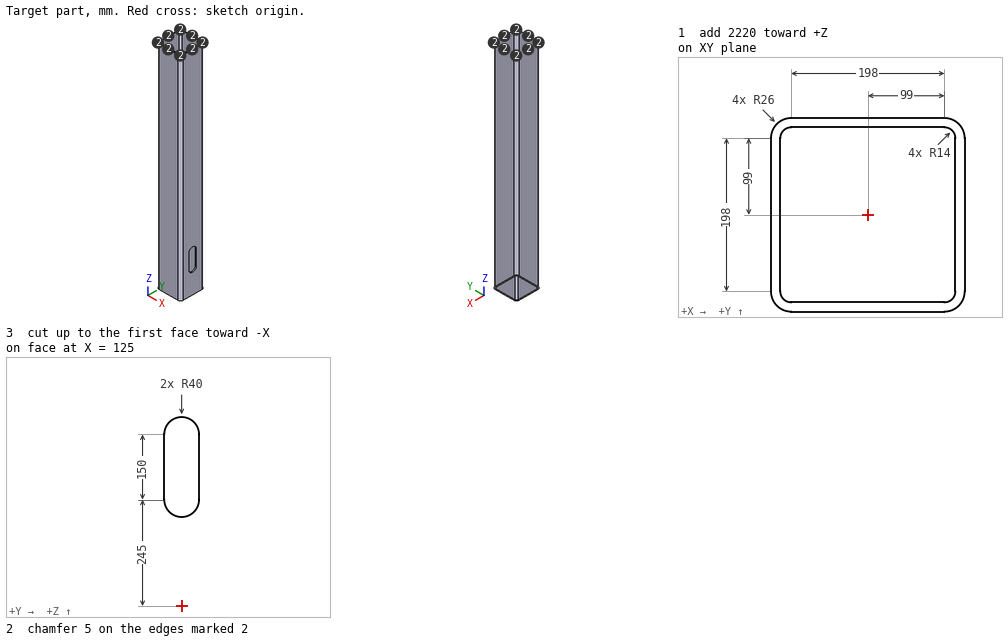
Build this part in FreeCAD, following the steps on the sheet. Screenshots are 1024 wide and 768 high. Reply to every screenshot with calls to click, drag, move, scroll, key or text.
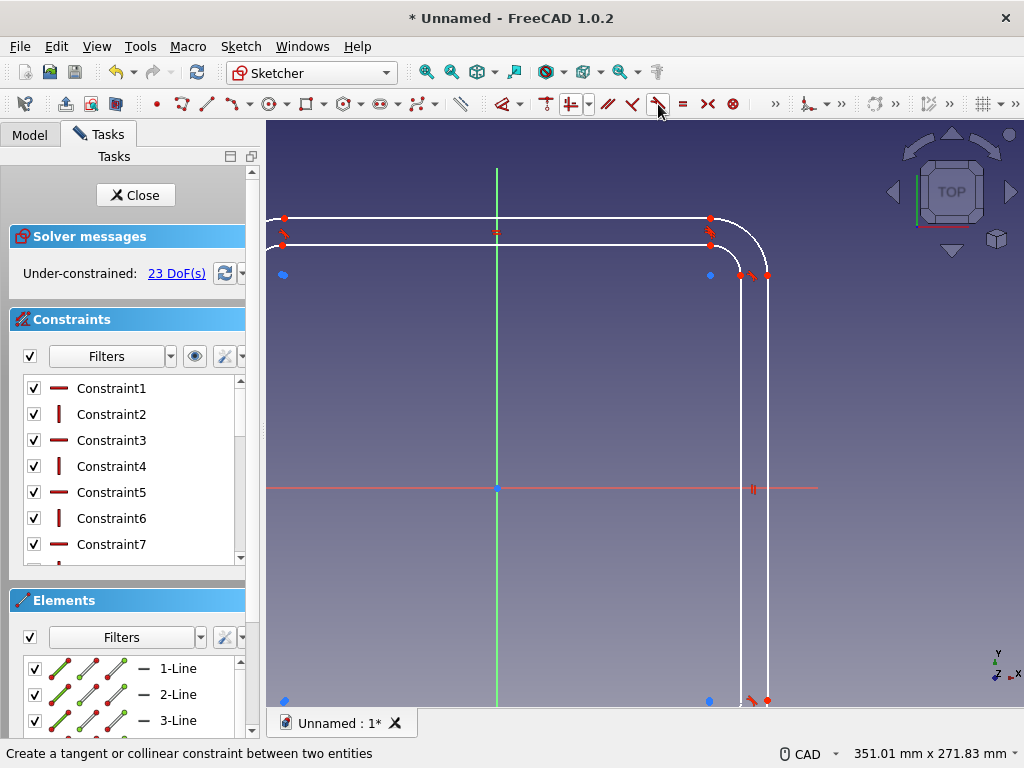
click(411, 245)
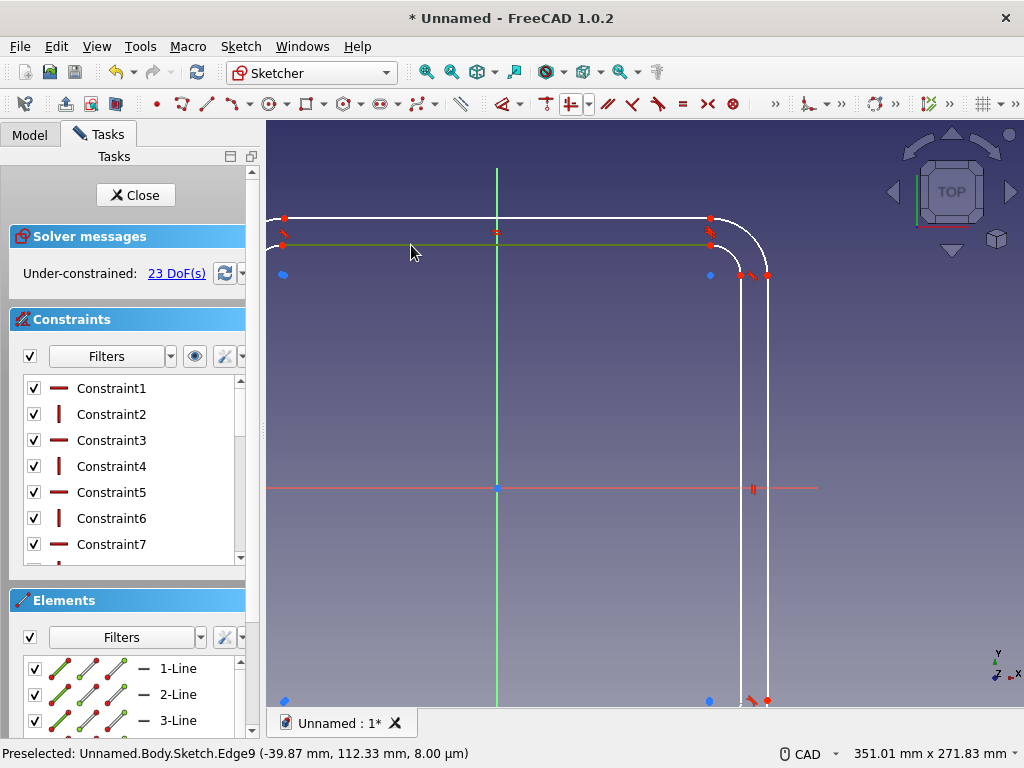
scroll(738, 262, down, 2)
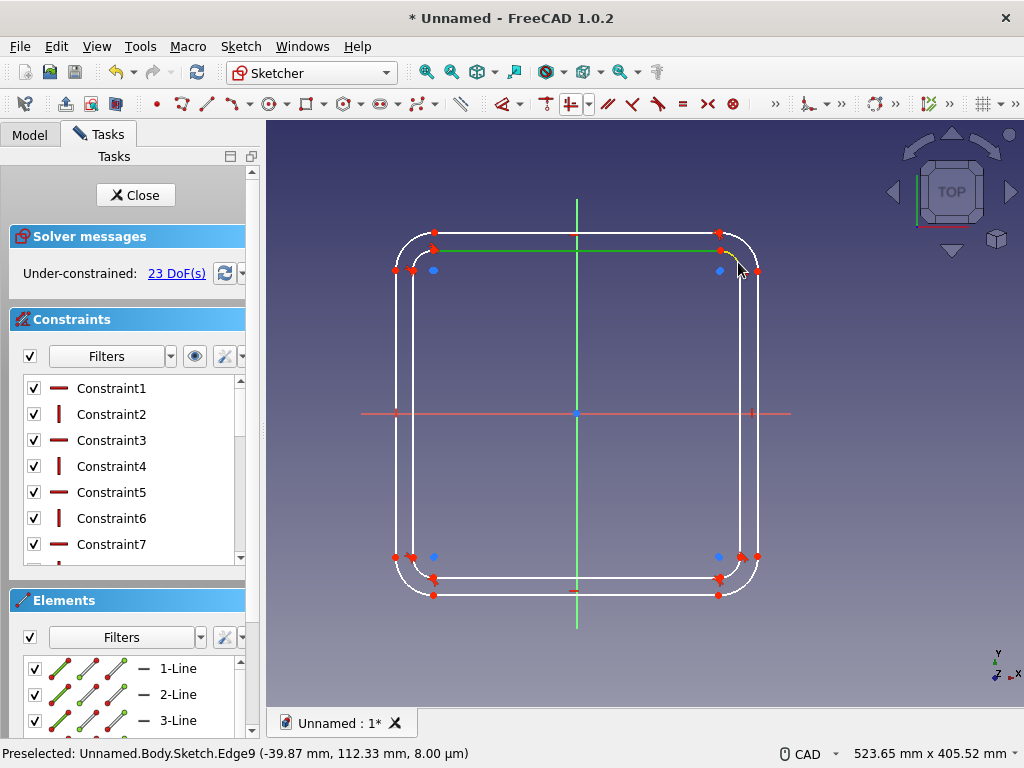
scroll(424, 253, up, 2)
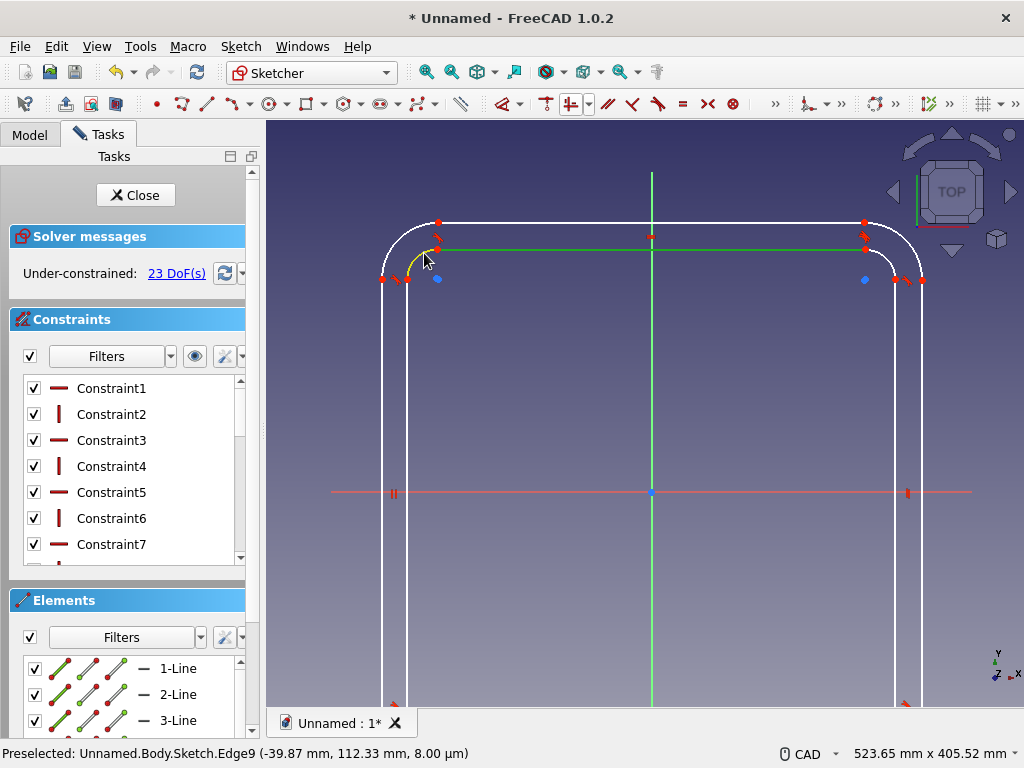
click(424, 253)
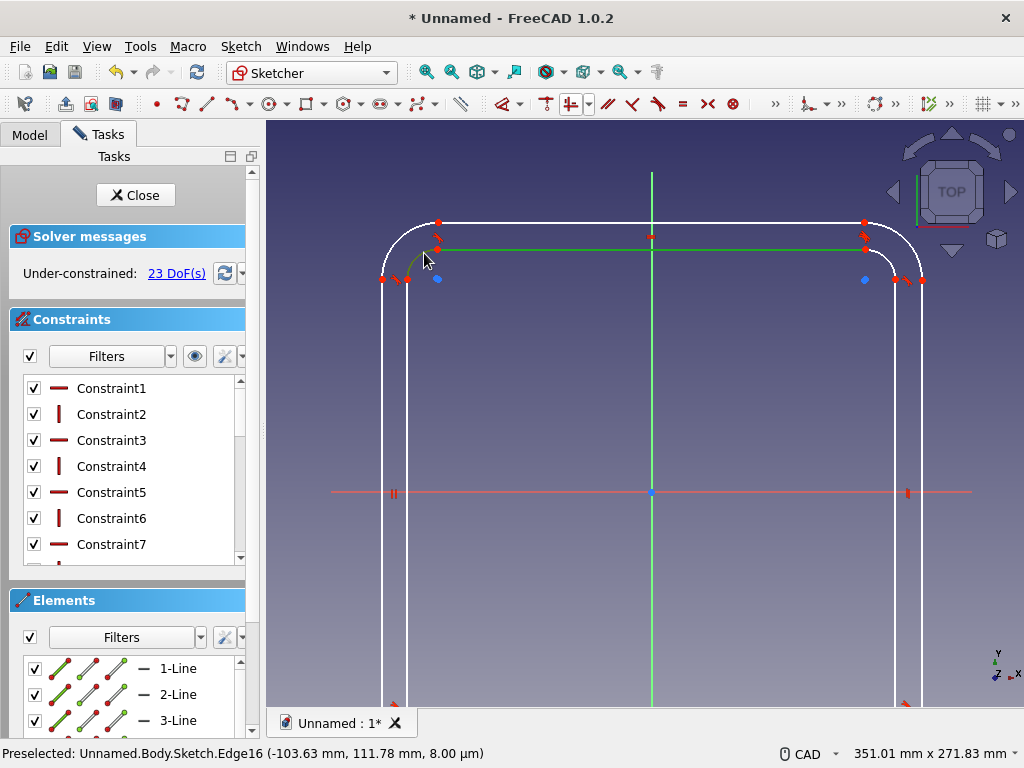
click(658, 104)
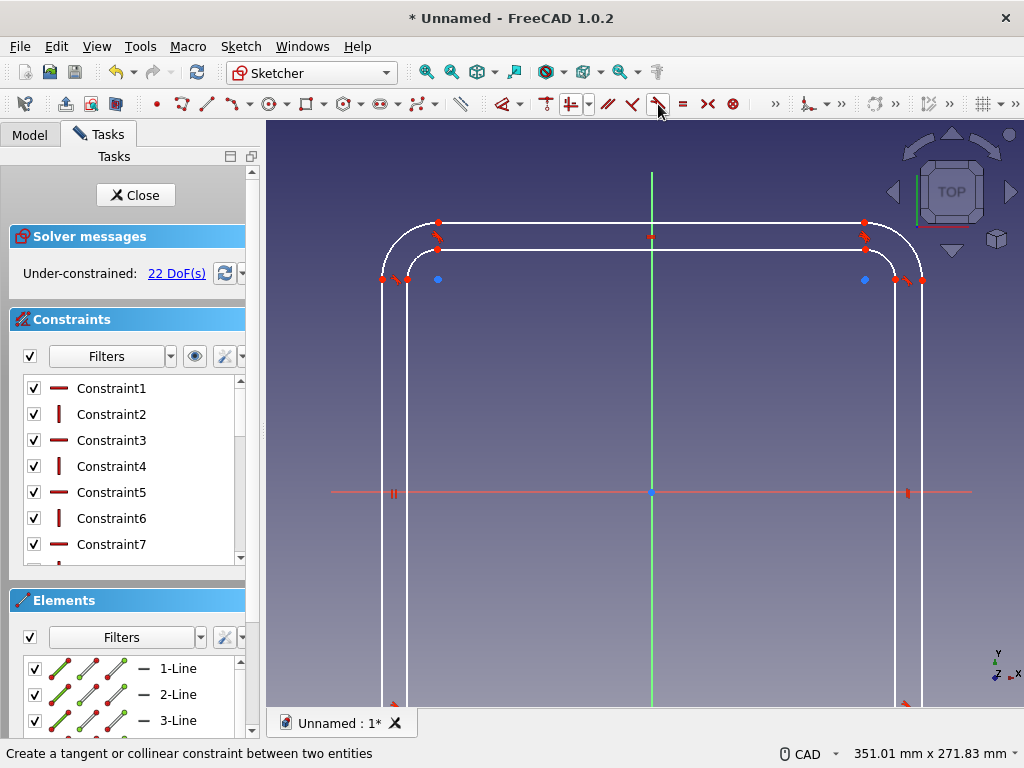
scroll(424, 253, down, 2)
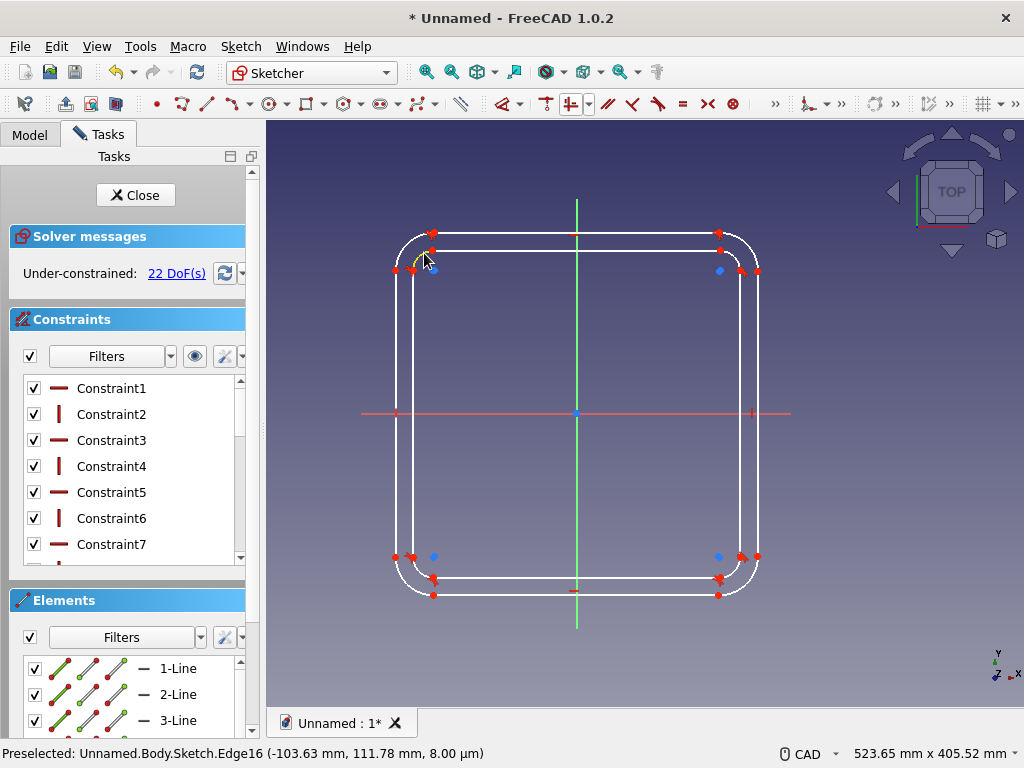
click(740, 357)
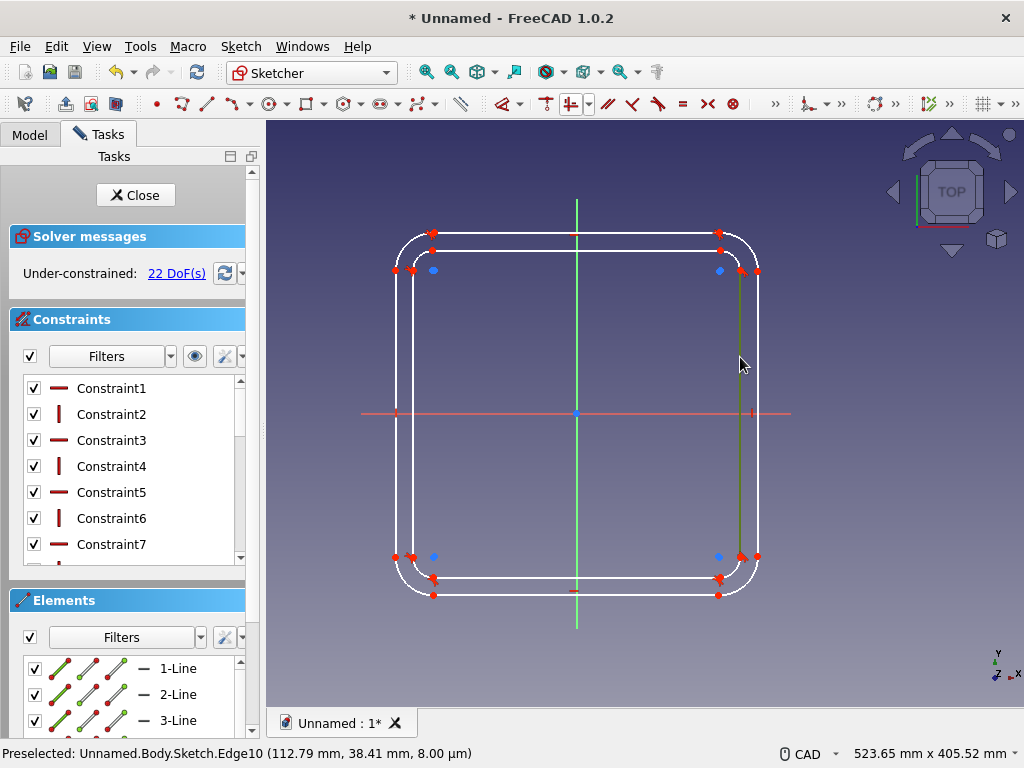
scroll(738, 262, up, 2)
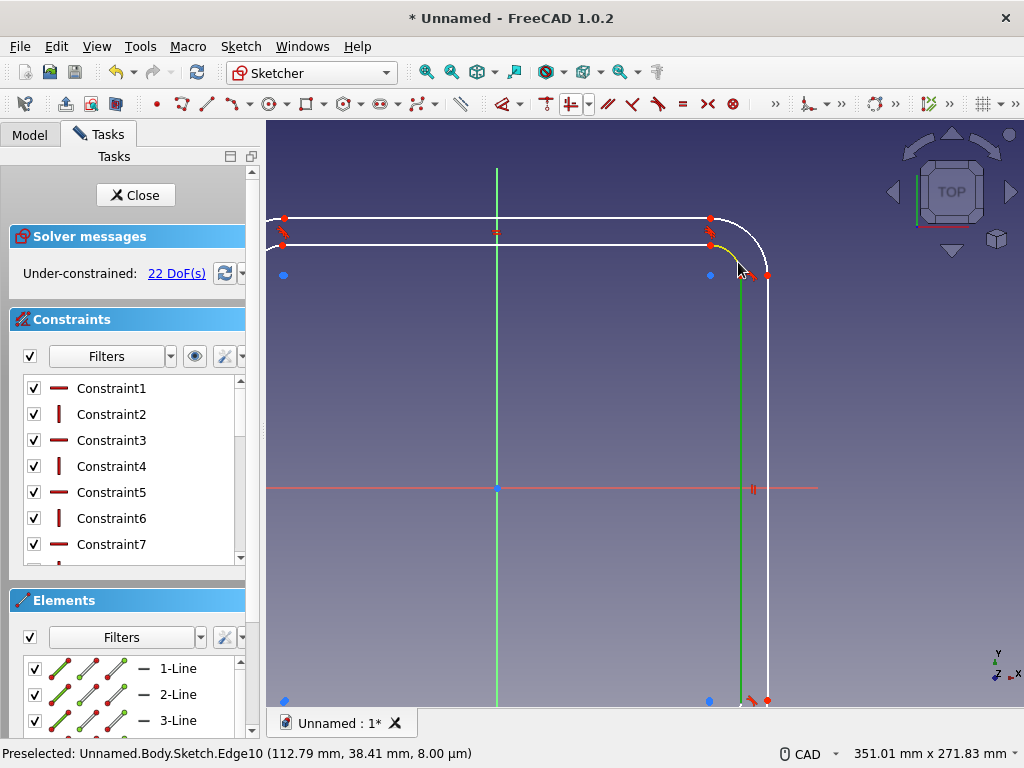
click(737, 262)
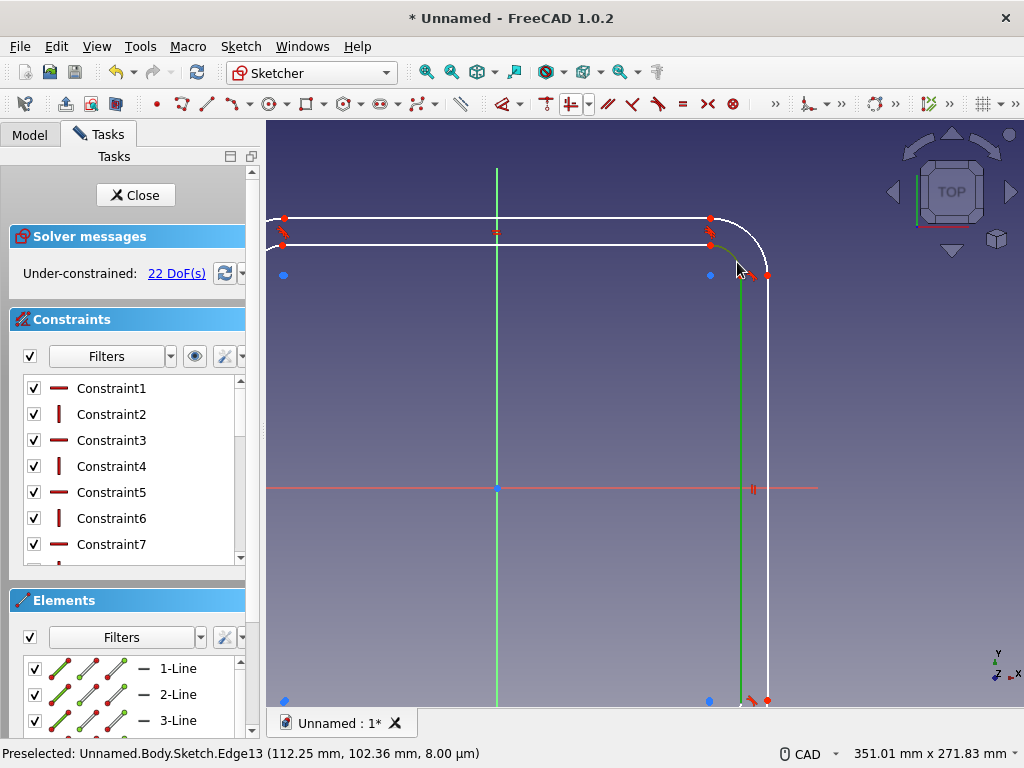
click(658, 104)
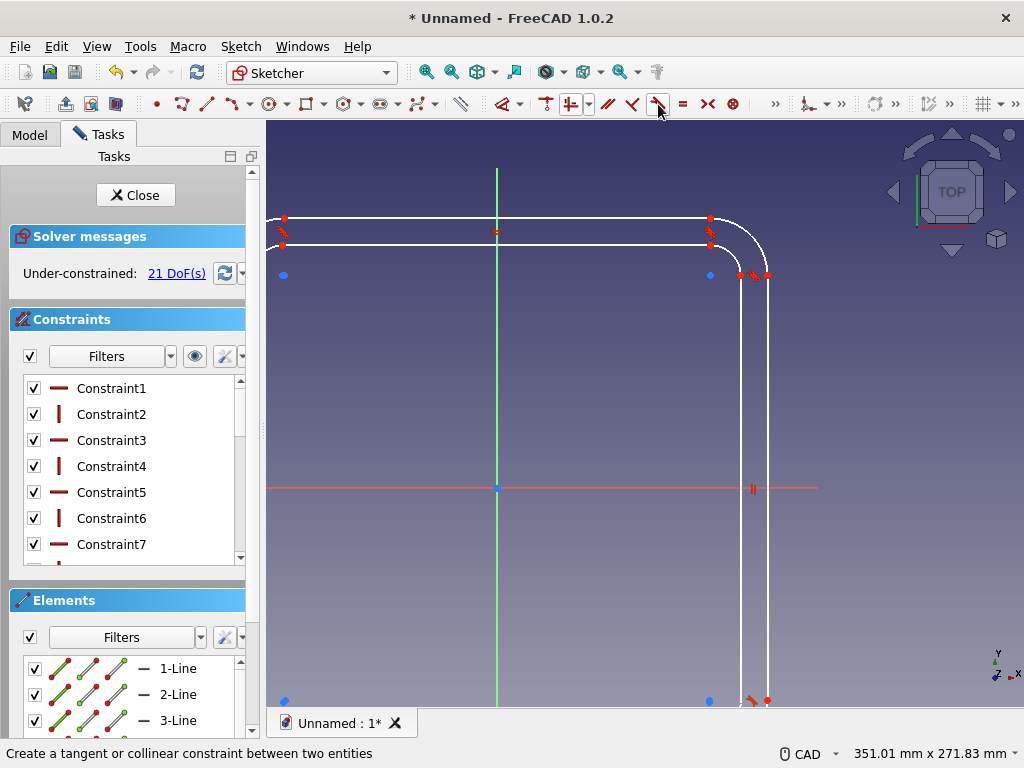
click(741, 404)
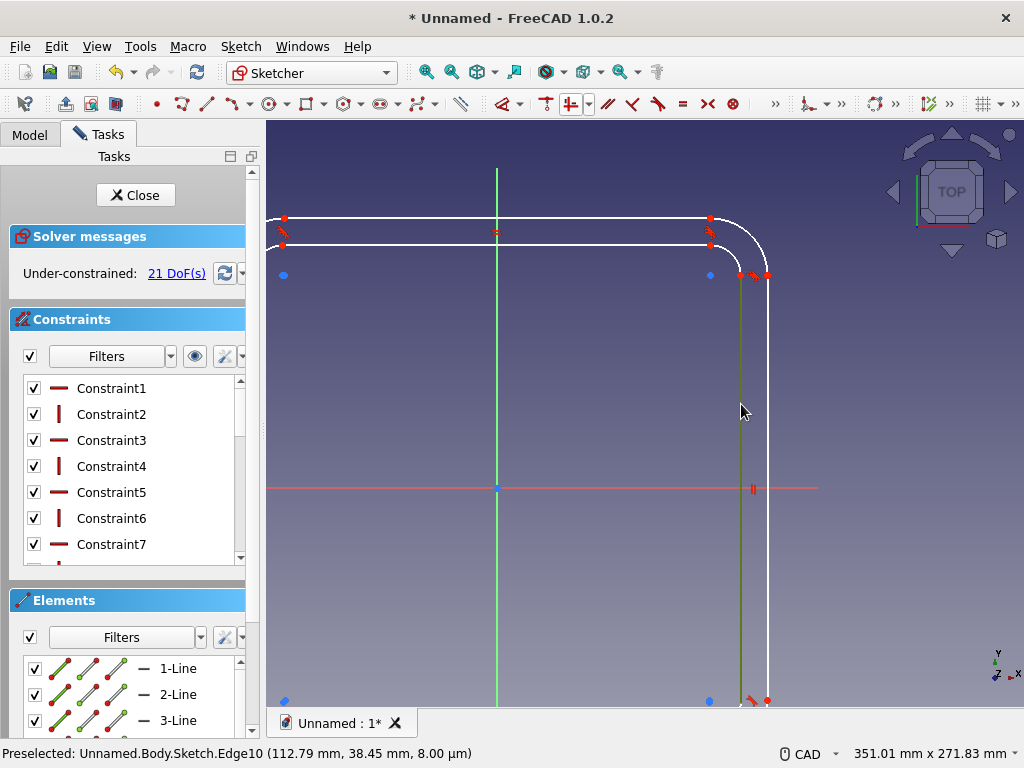
scroll(738, 262, down, 2)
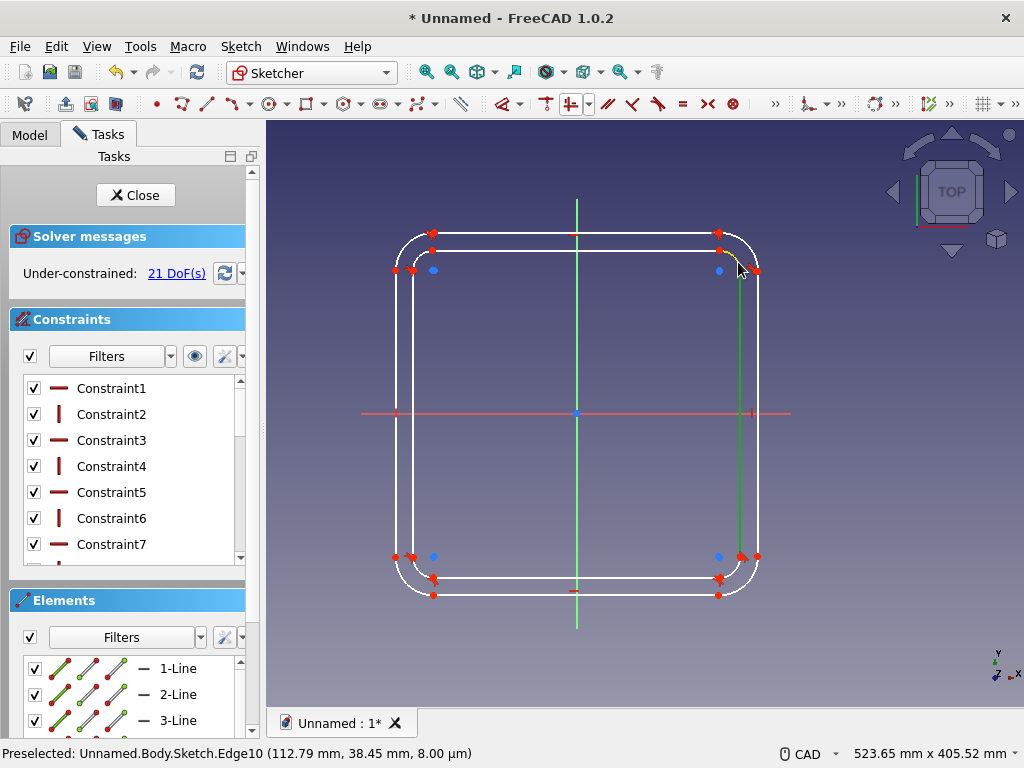
scroll(729, 576, up, 2)